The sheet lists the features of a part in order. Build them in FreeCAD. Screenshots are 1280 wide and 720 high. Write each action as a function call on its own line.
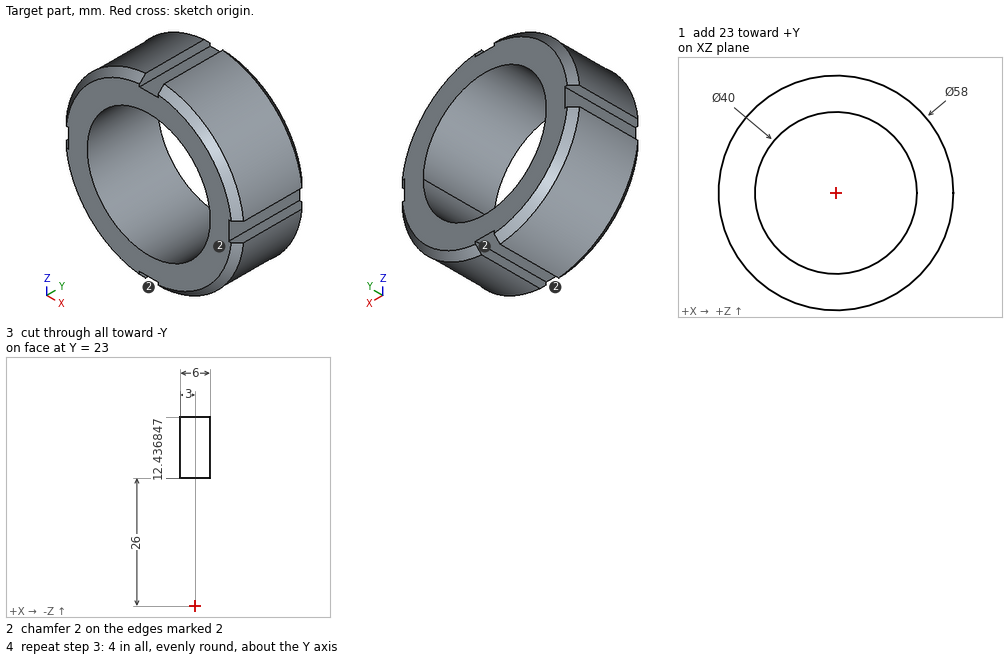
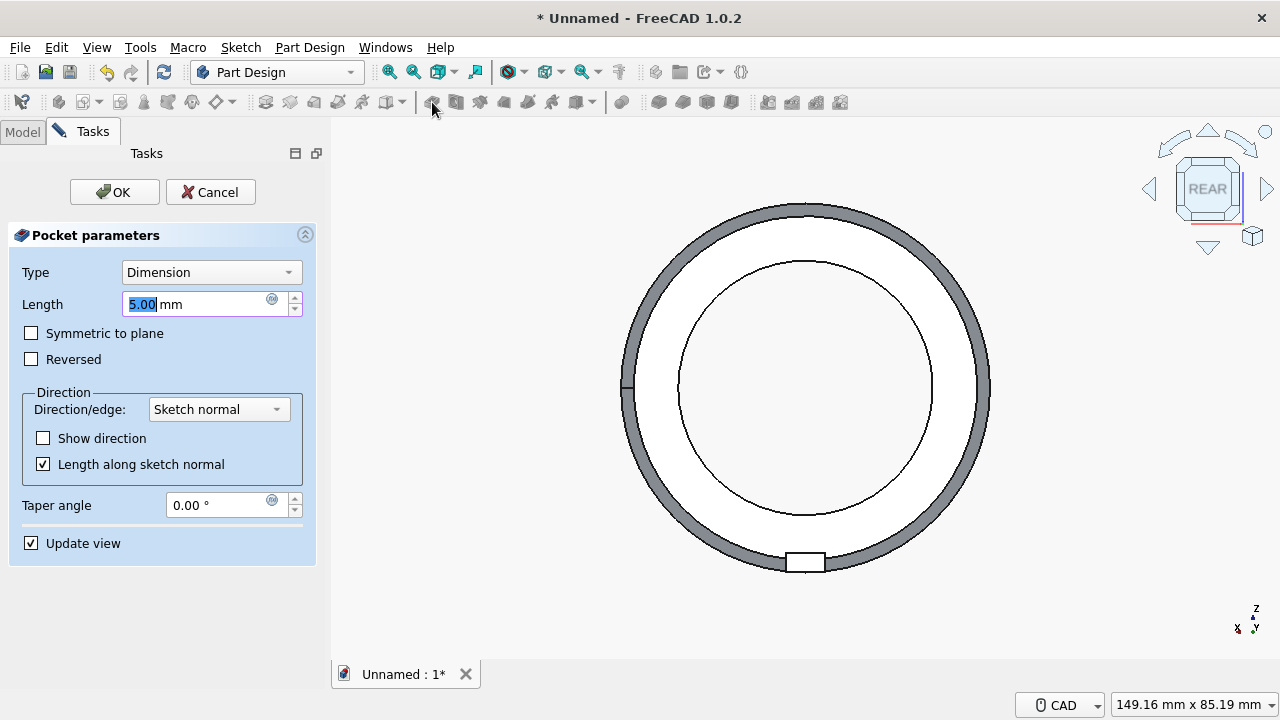
click(212, 272)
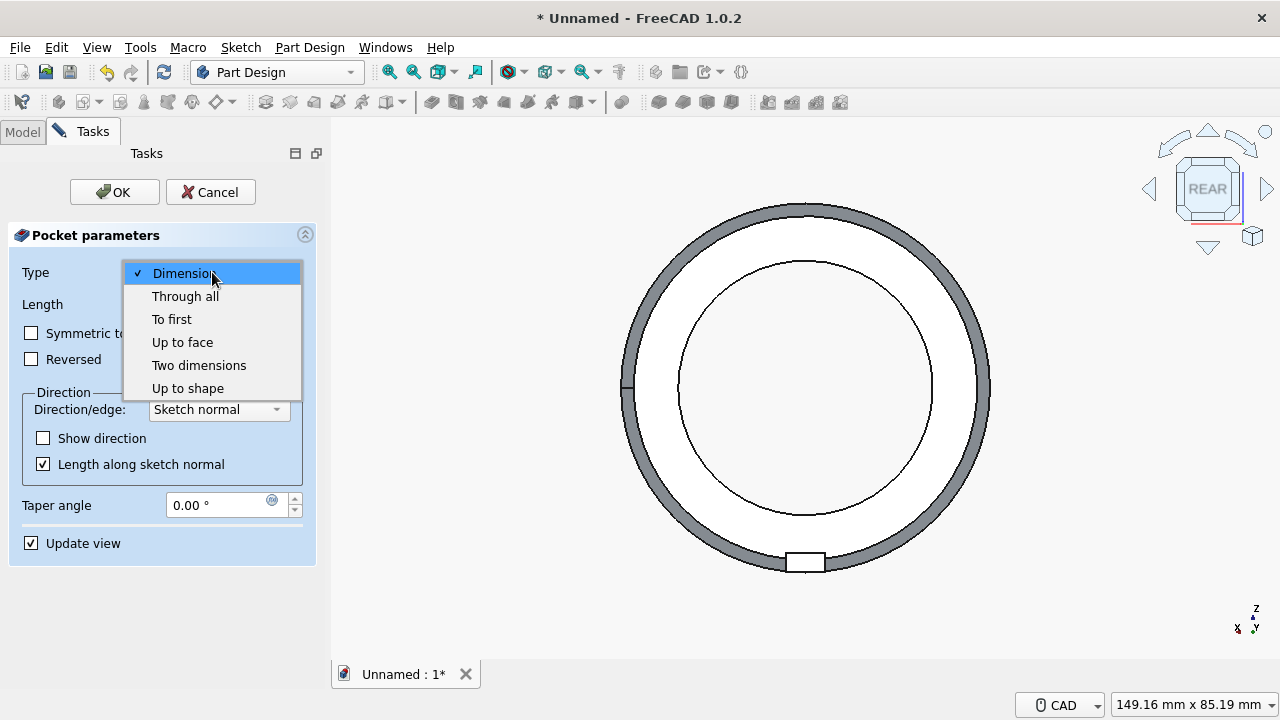
click(212, 296)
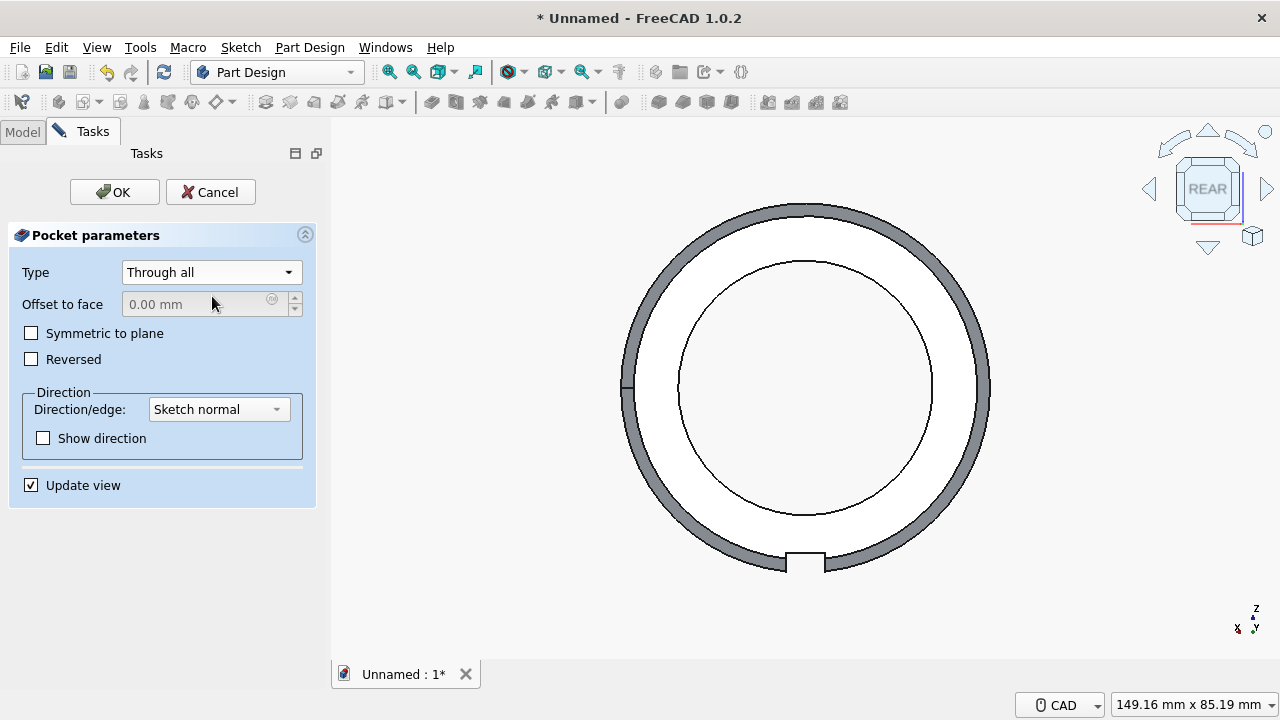
click(115, 192)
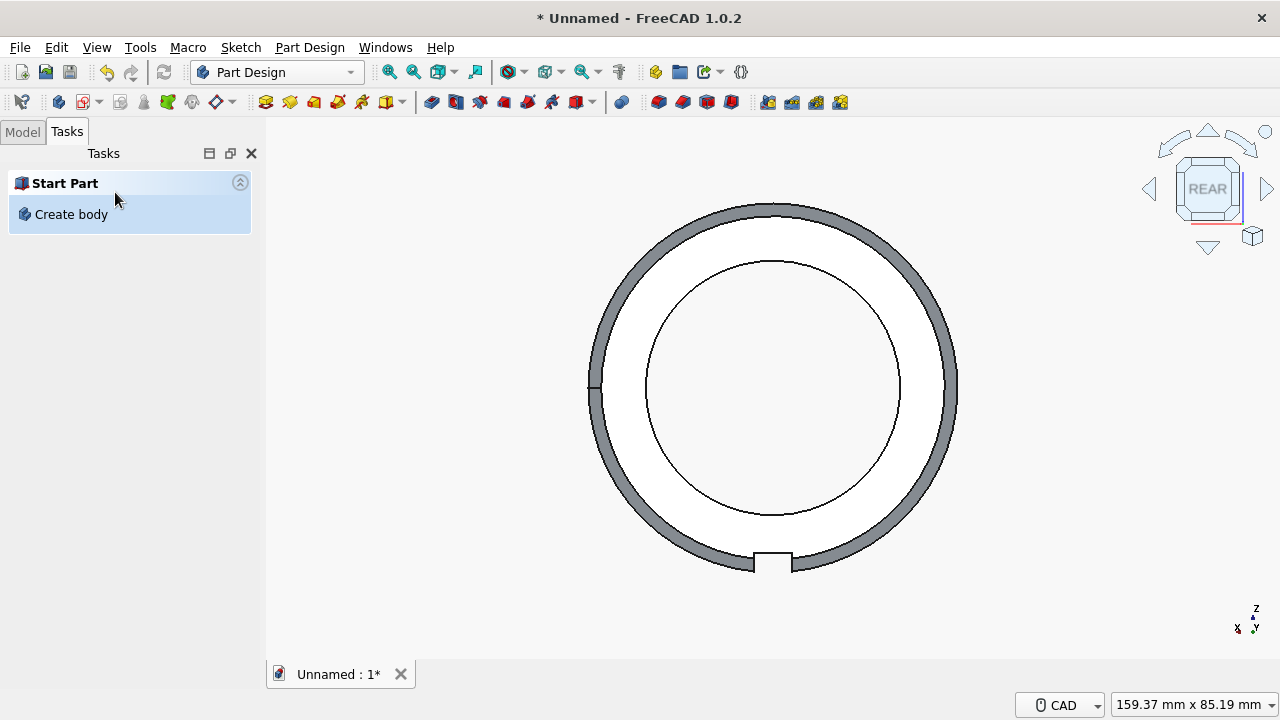
click(23, 131)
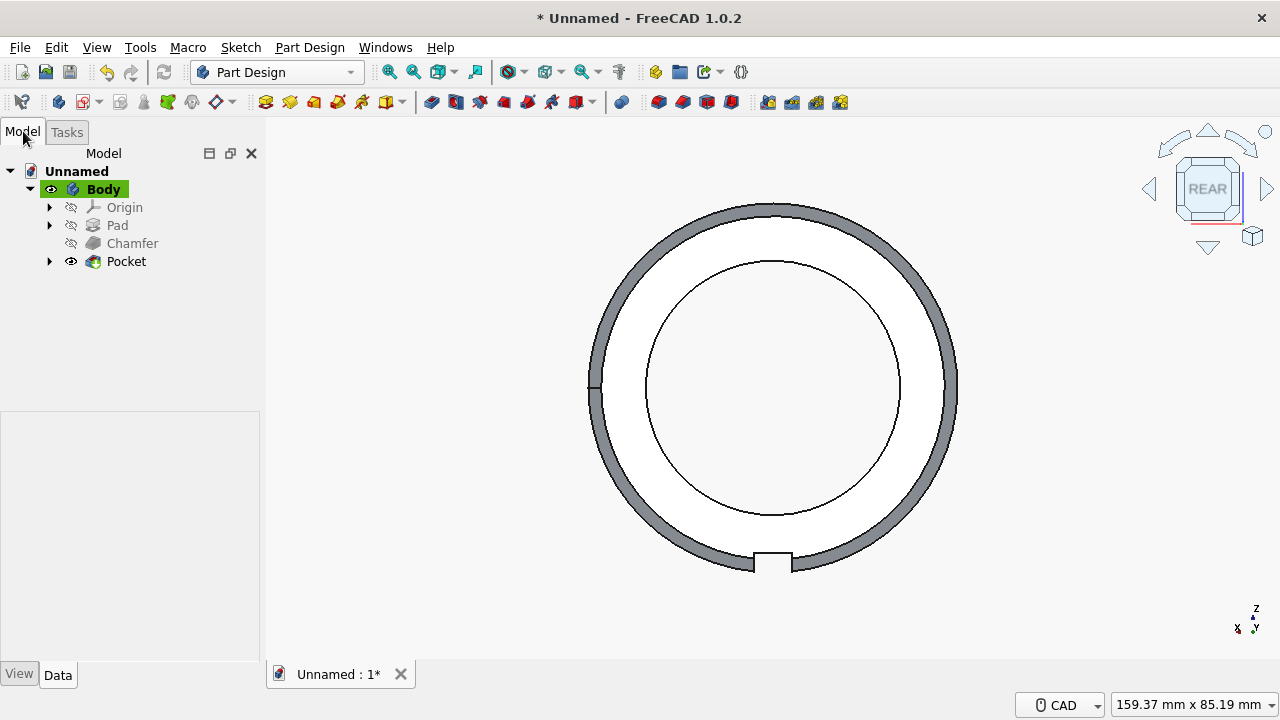
click(116, 261)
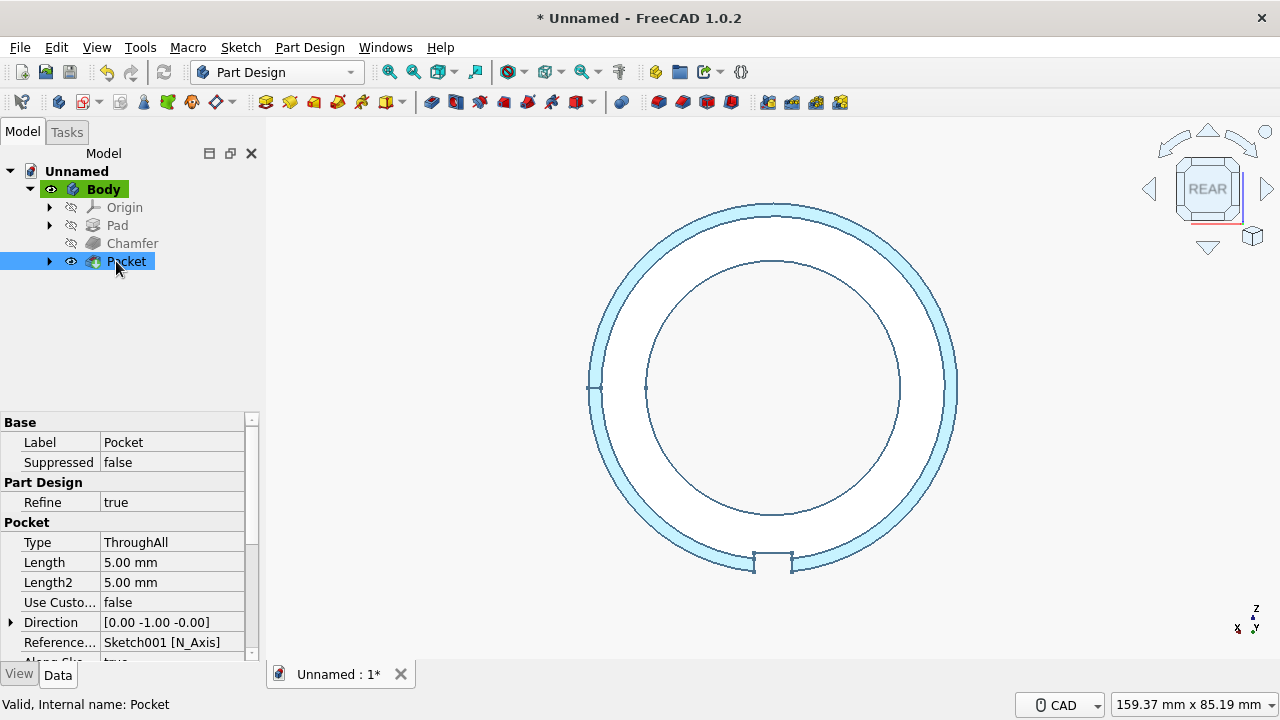
click(816, 102)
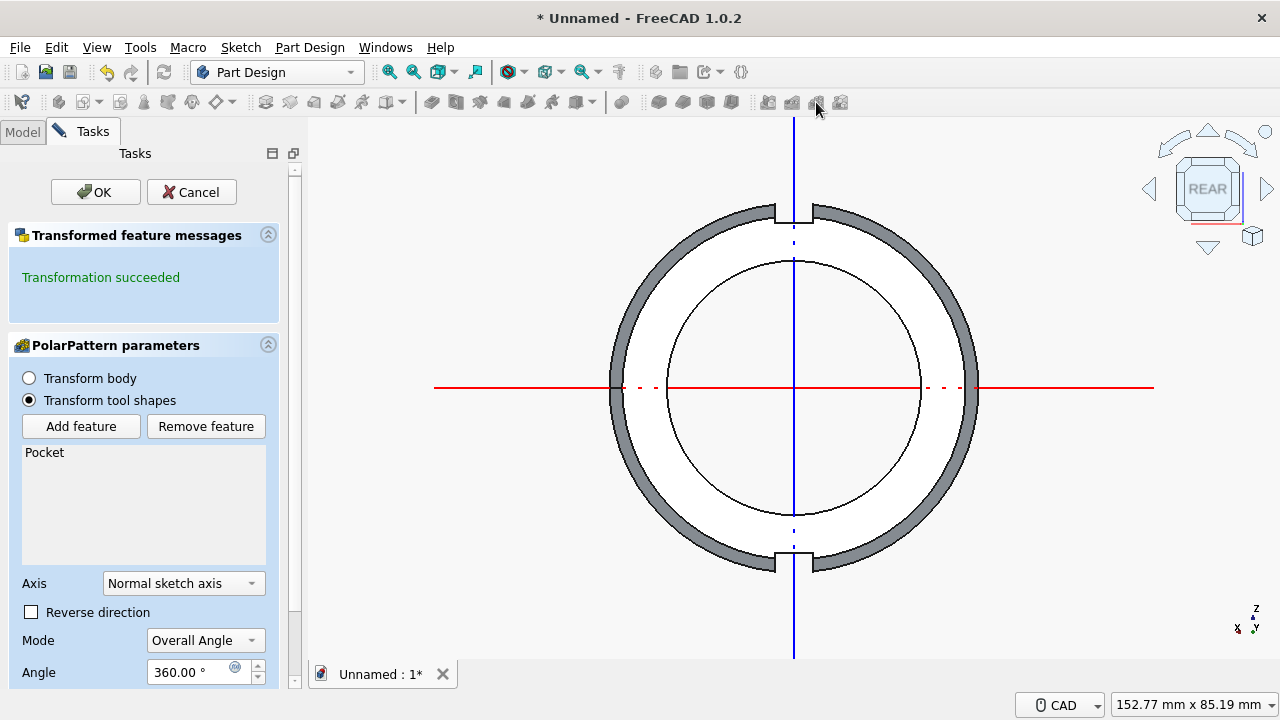
click(184, 584)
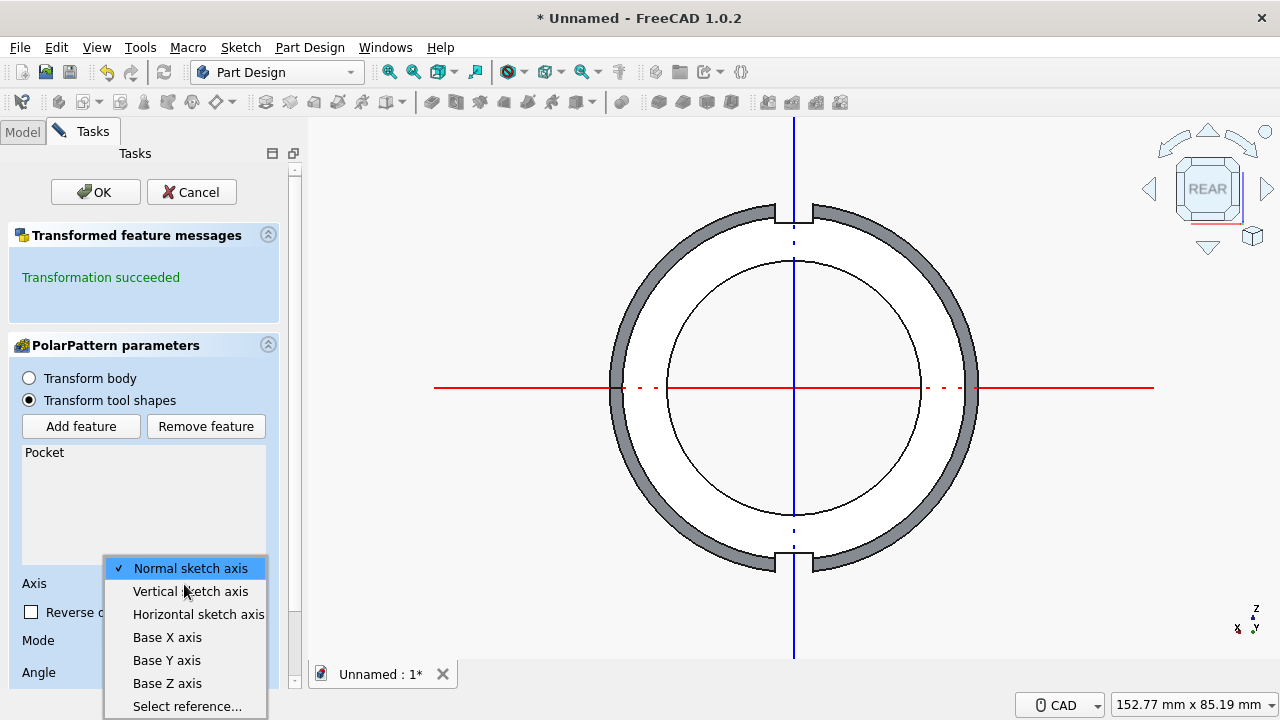
click(184, 660)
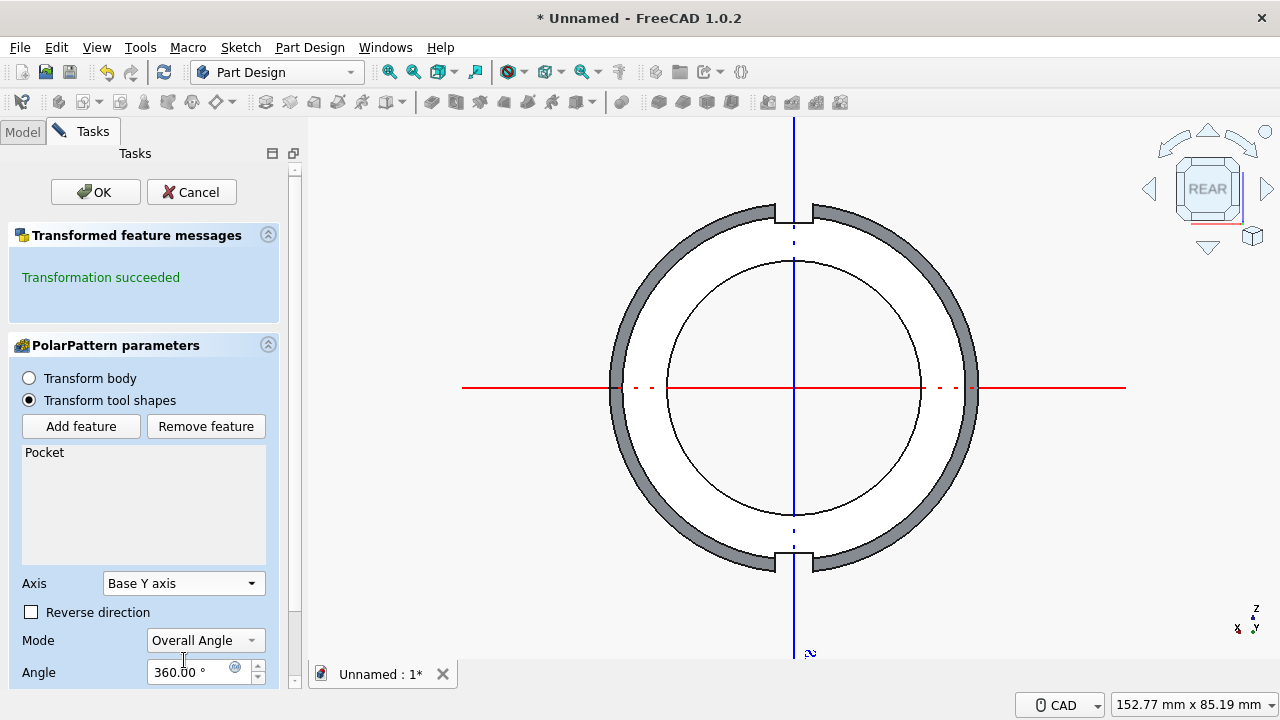
scroll(295, 426, down, 2)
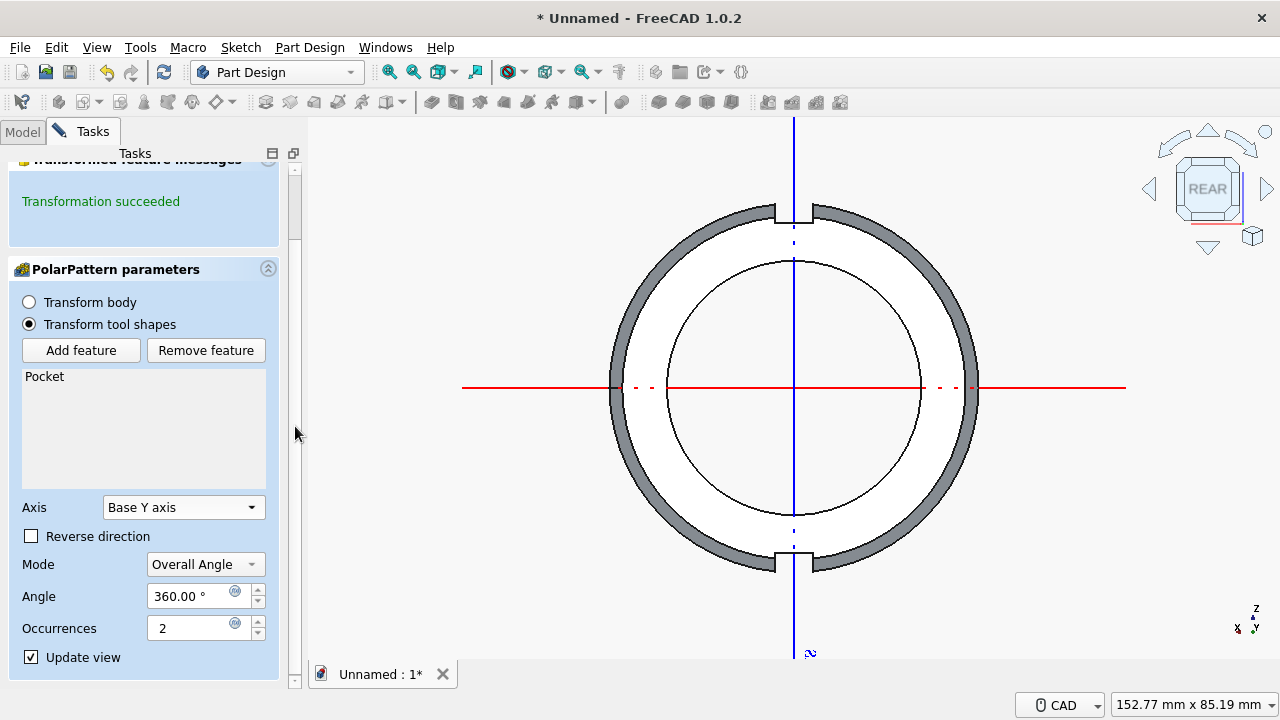
triple_click(198, 628)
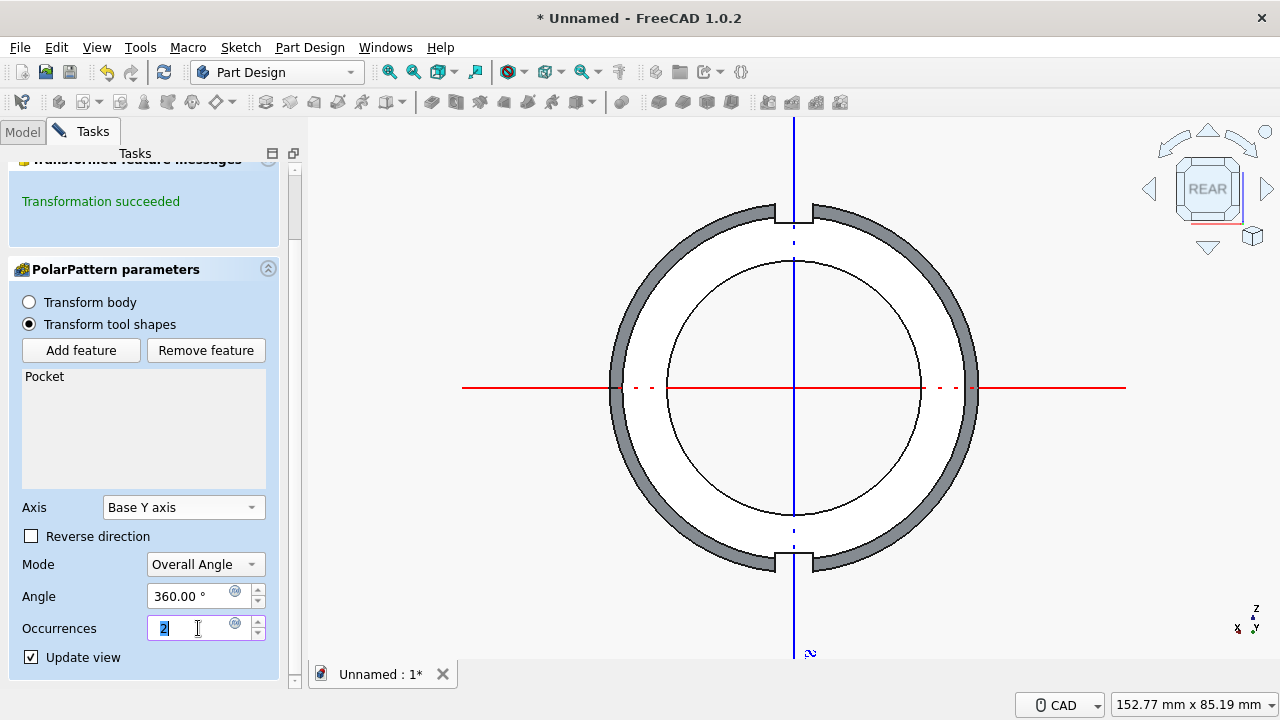
text(4)
key(Tab)